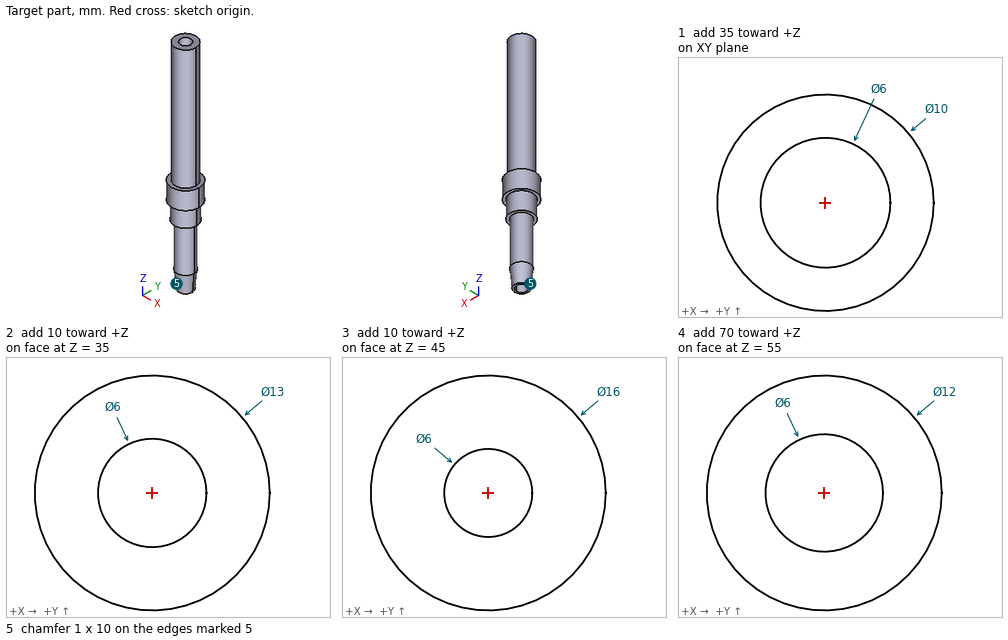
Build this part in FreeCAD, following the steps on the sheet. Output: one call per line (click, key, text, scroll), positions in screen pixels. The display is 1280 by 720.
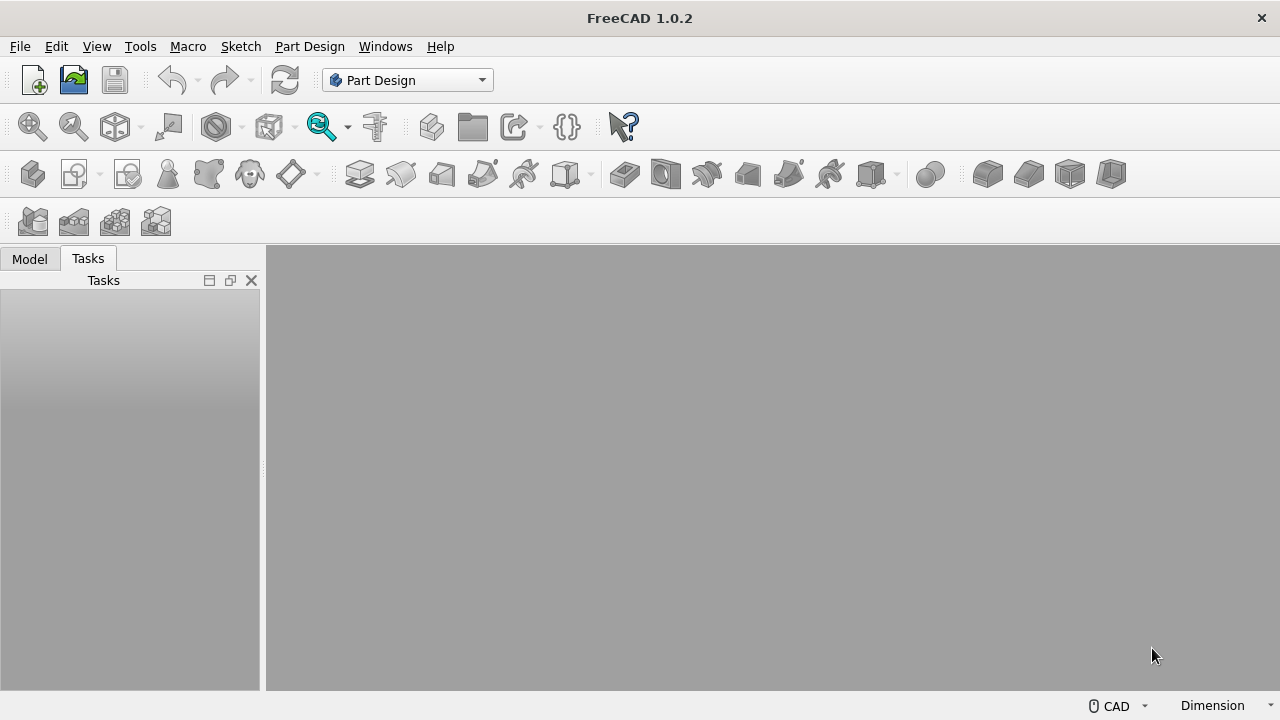
click(33, 80)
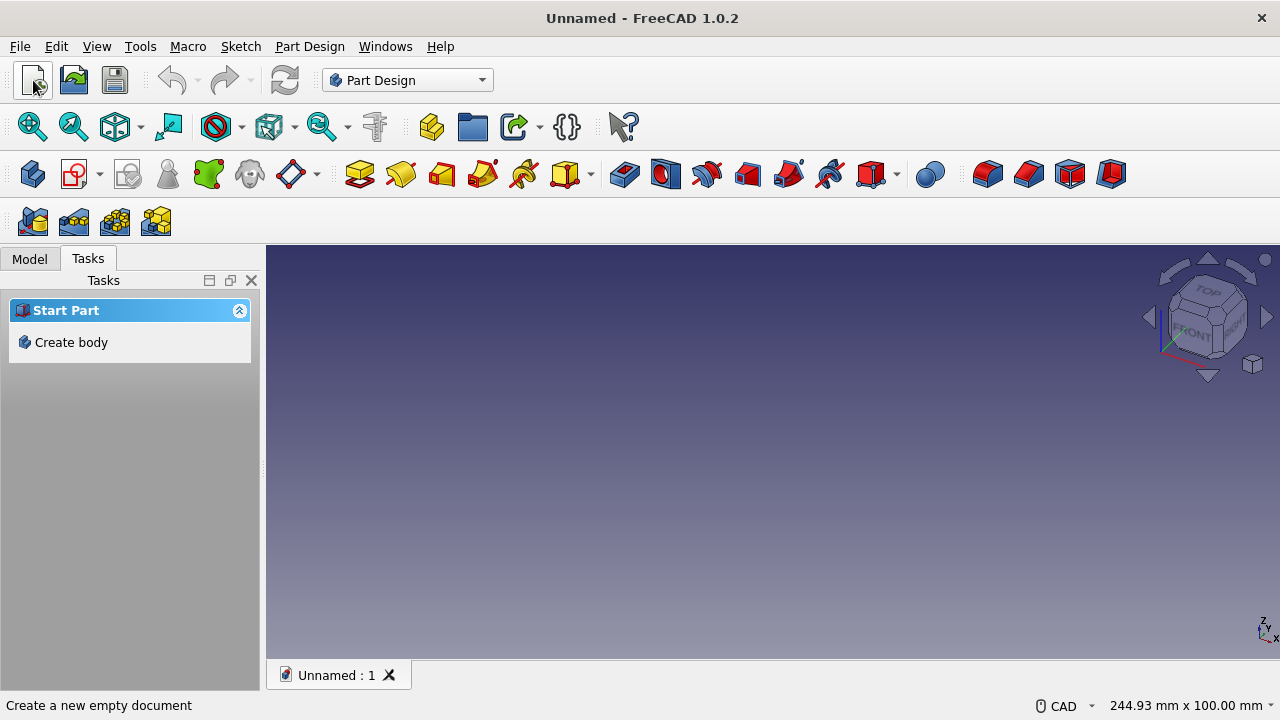
click(74, 174)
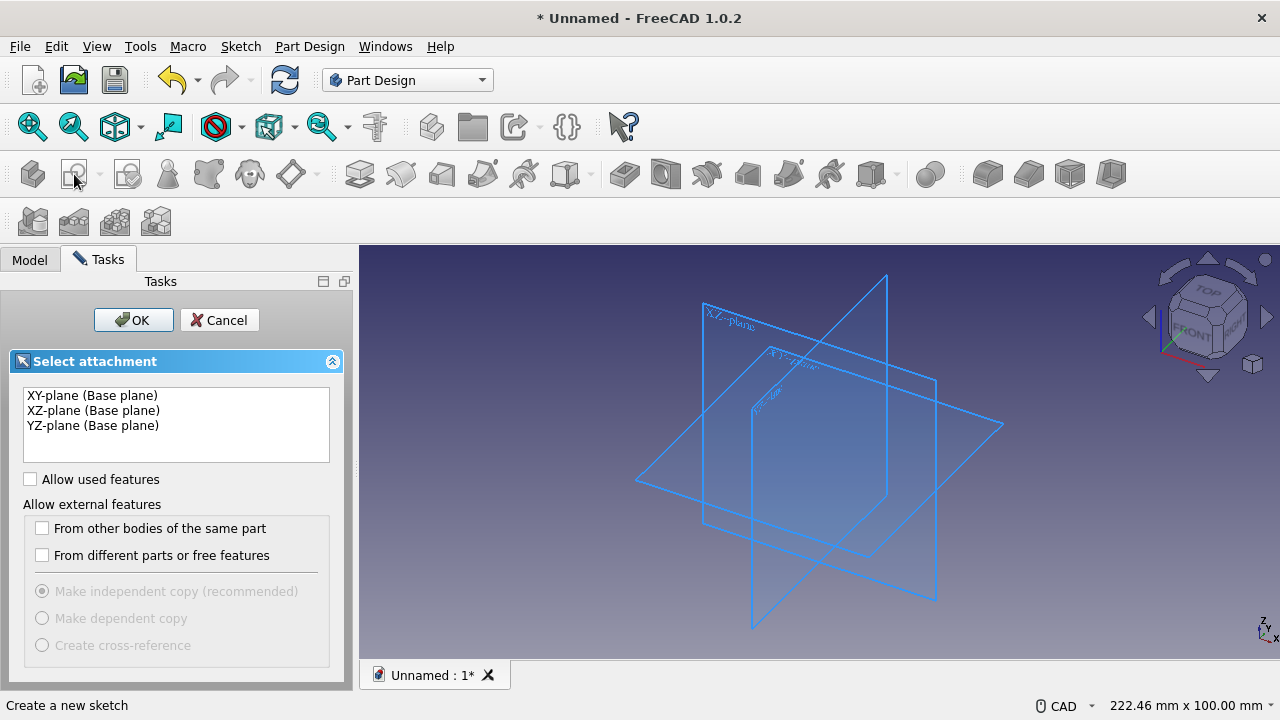
click(84, 396)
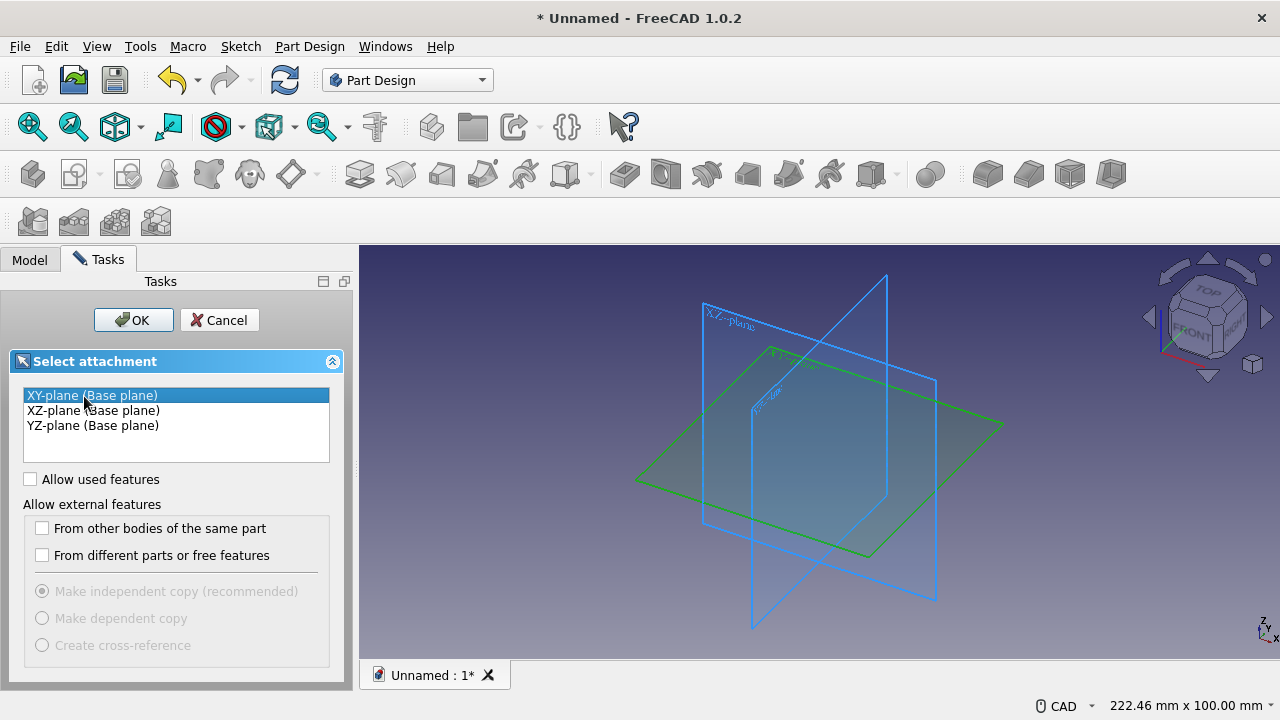
click(134, 320)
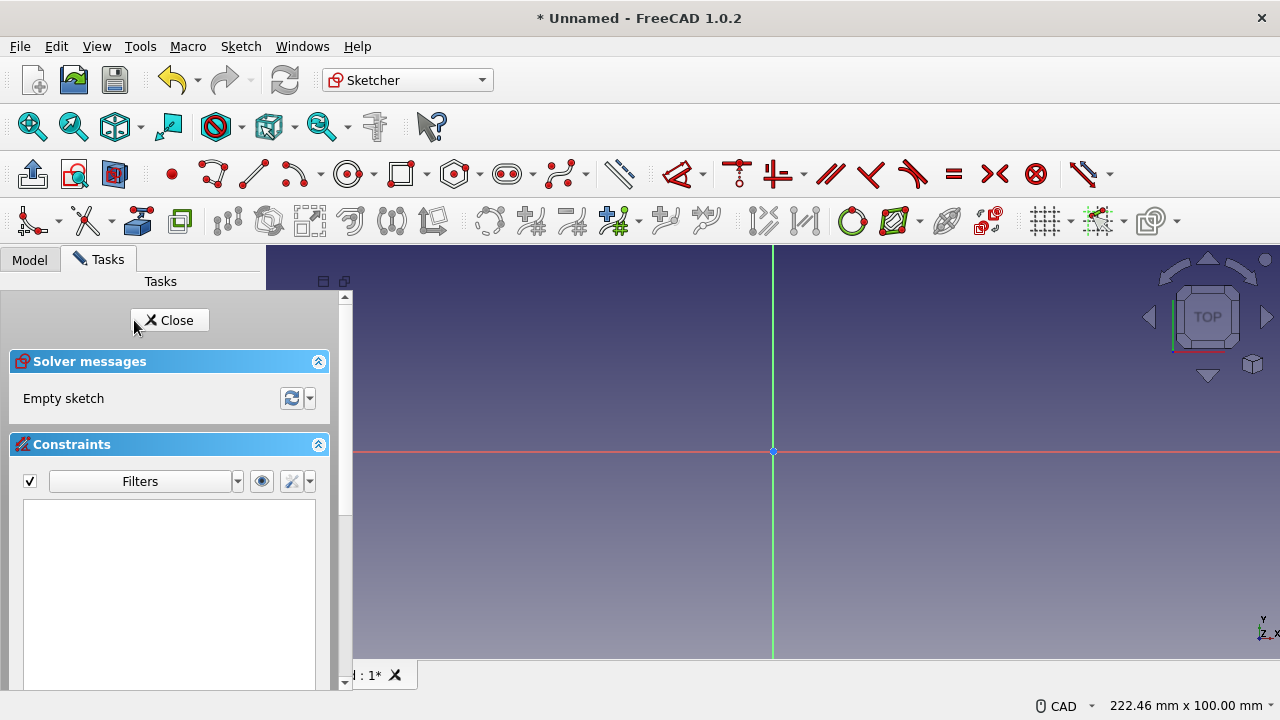
scroll(787, 452, up, 9)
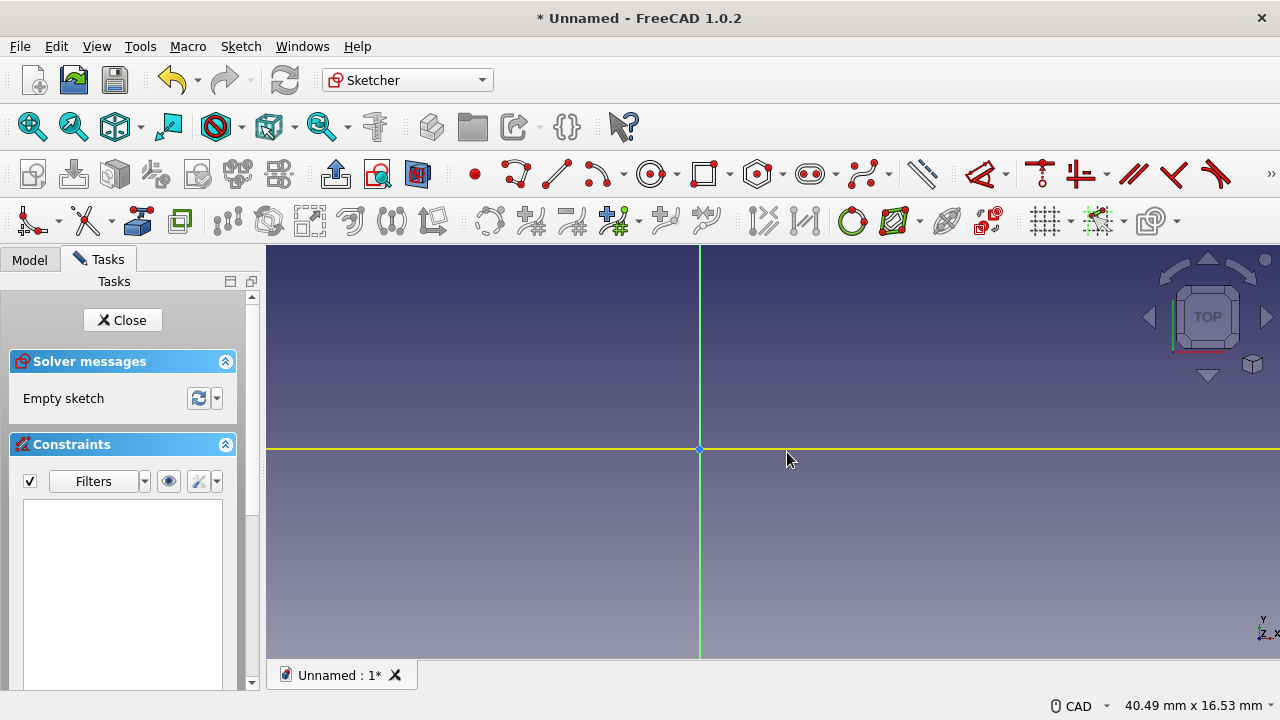
click(650, 174)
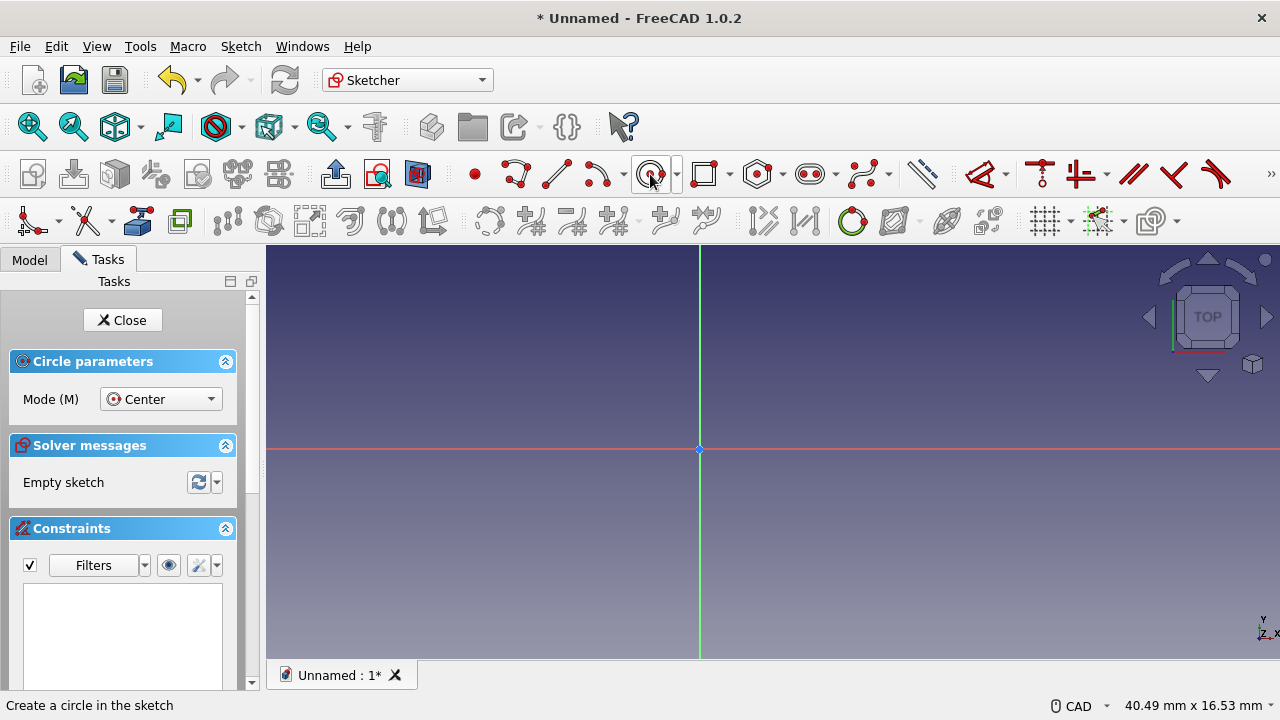
click(700, 449)
click(788, 361)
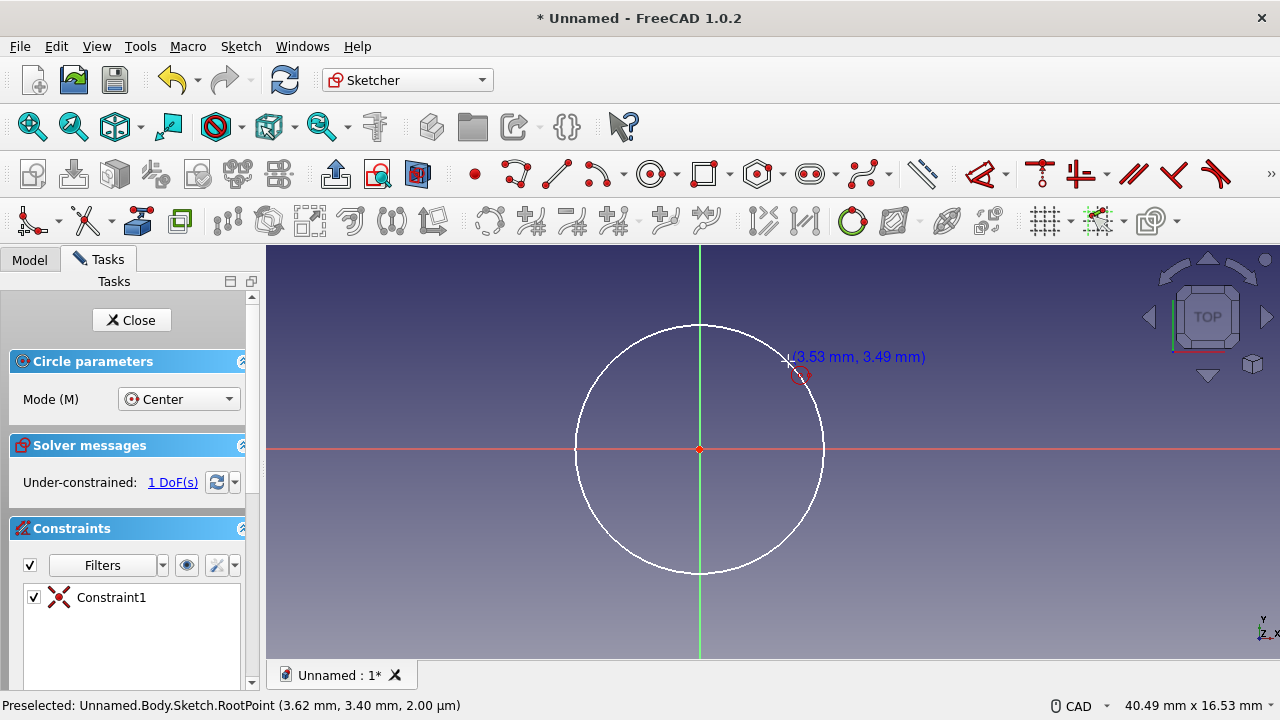
click(700, 449)
click(753, 396)
key(Escape)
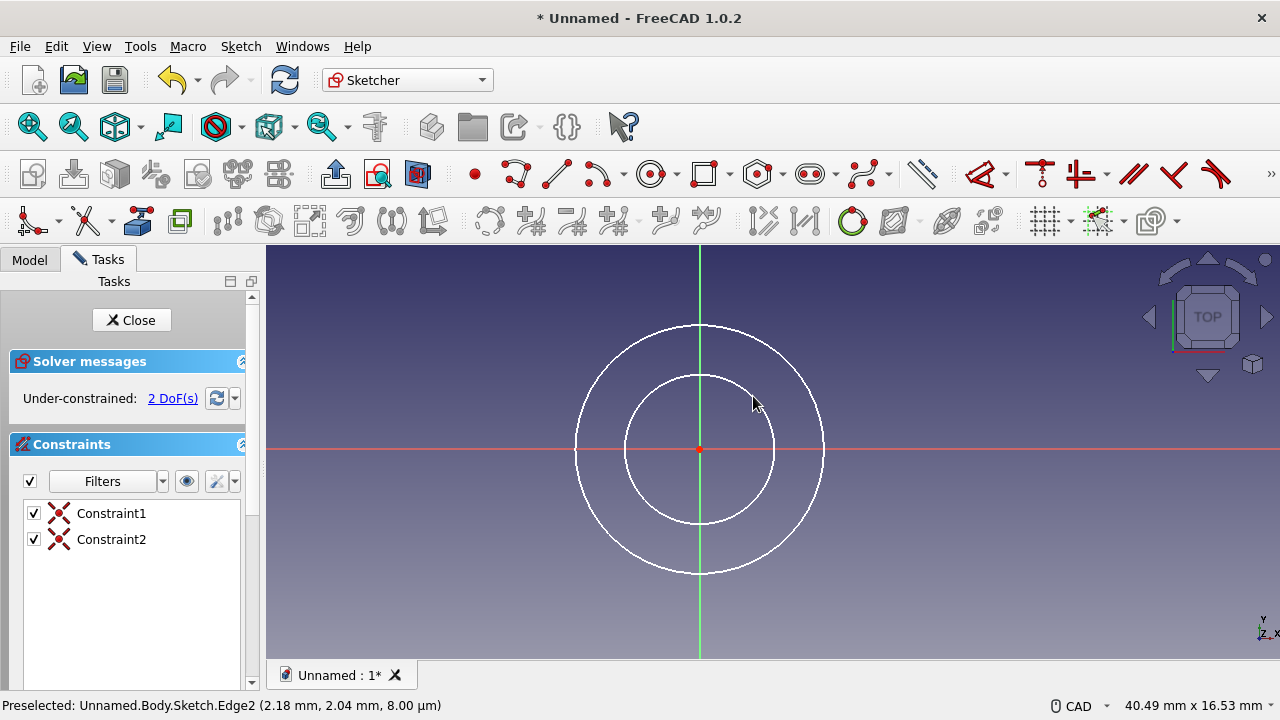
click(980, 174)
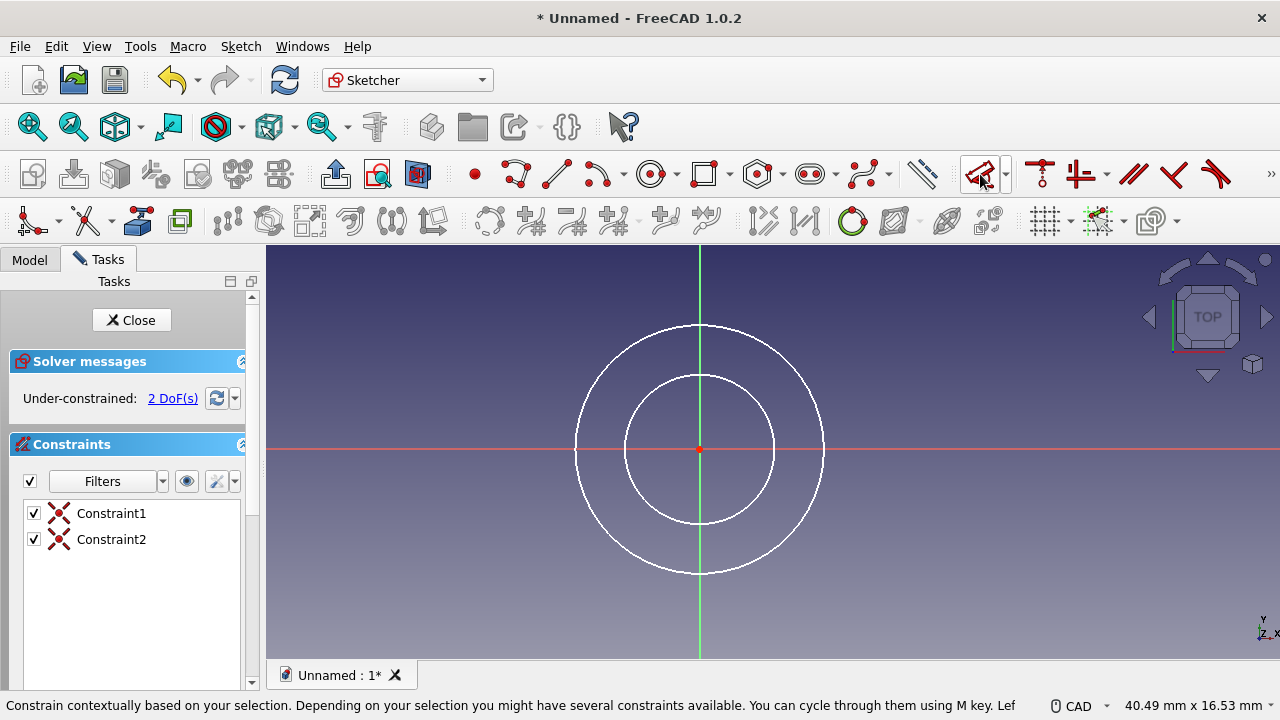
click(787, 361)
click(809, 338)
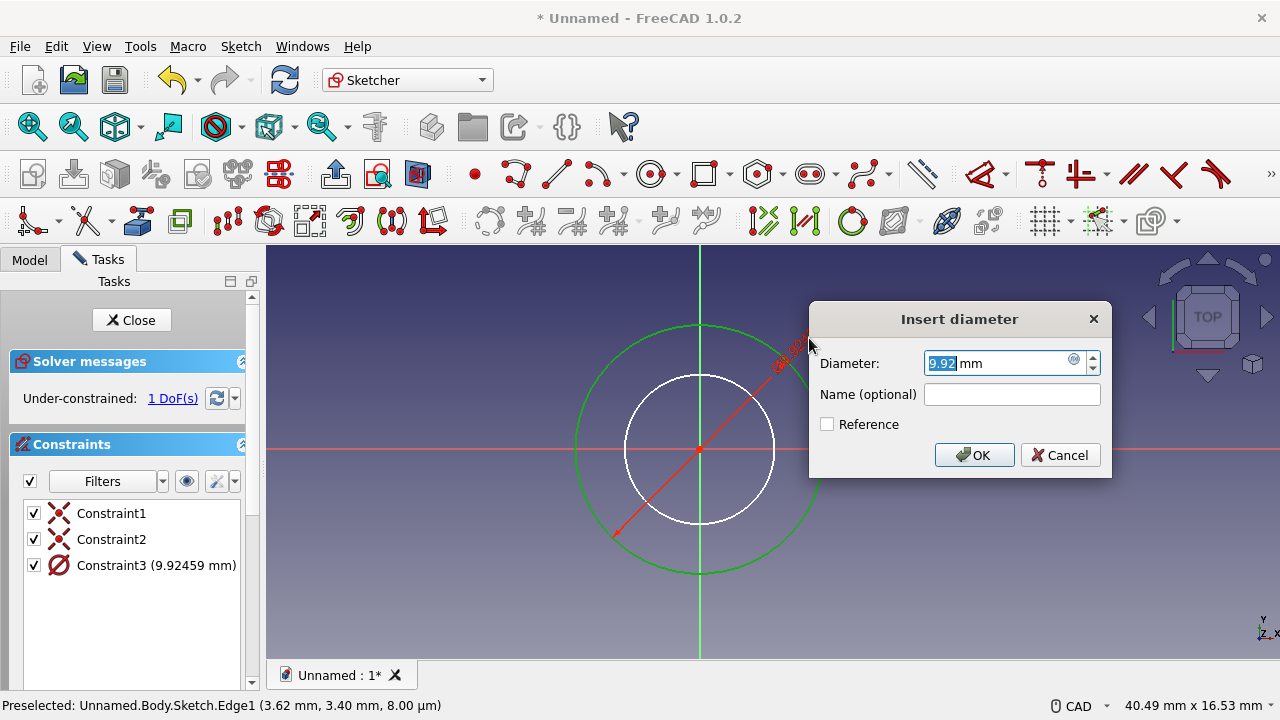
text(10)
key(Return)